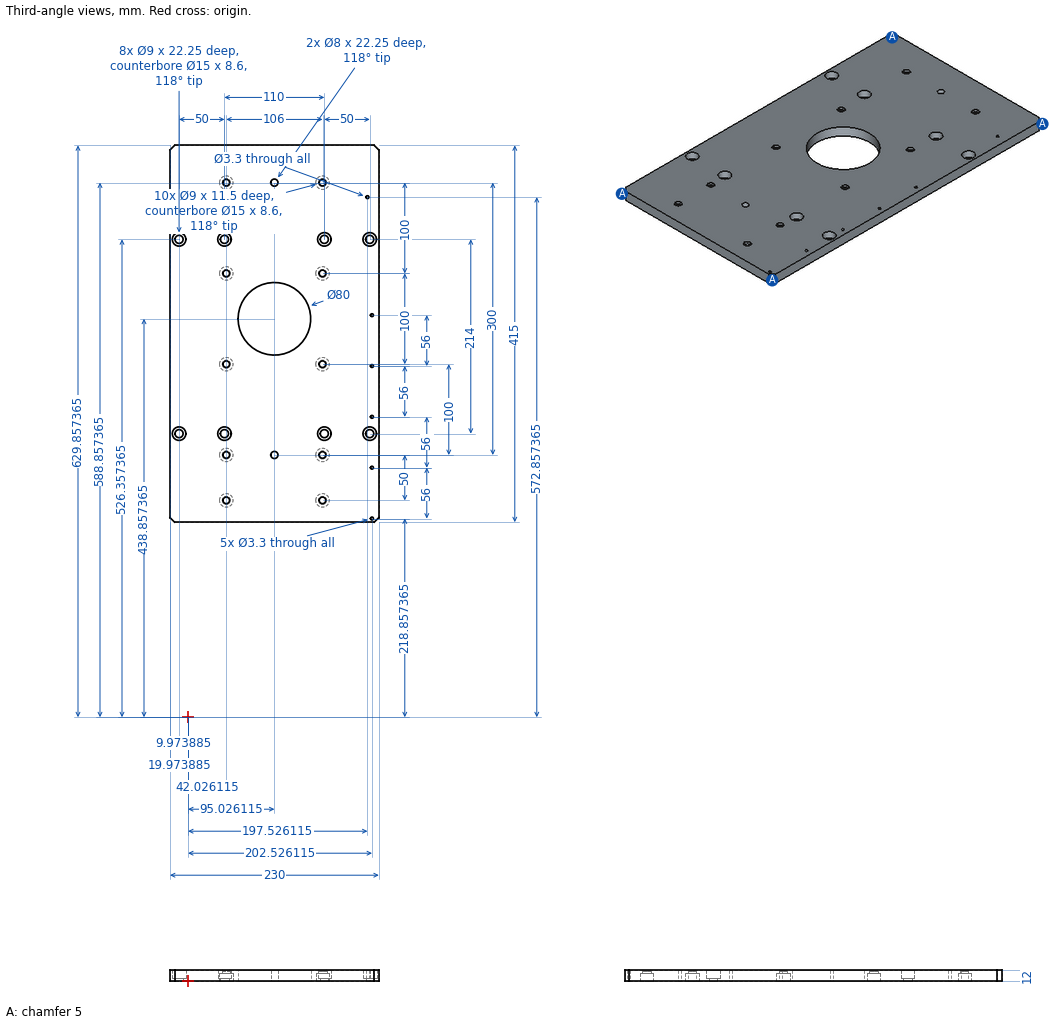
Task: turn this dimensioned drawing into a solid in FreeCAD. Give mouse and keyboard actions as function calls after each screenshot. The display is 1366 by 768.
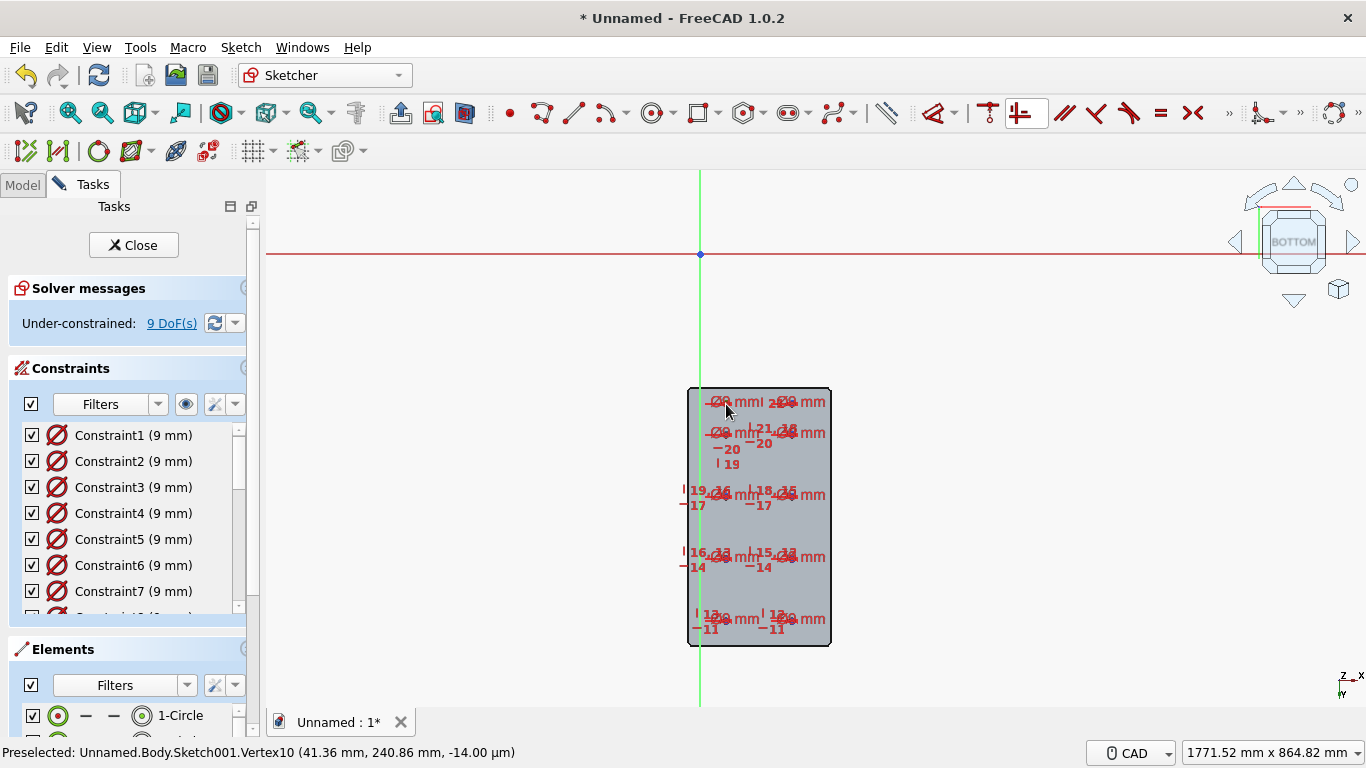
click(1042, 114)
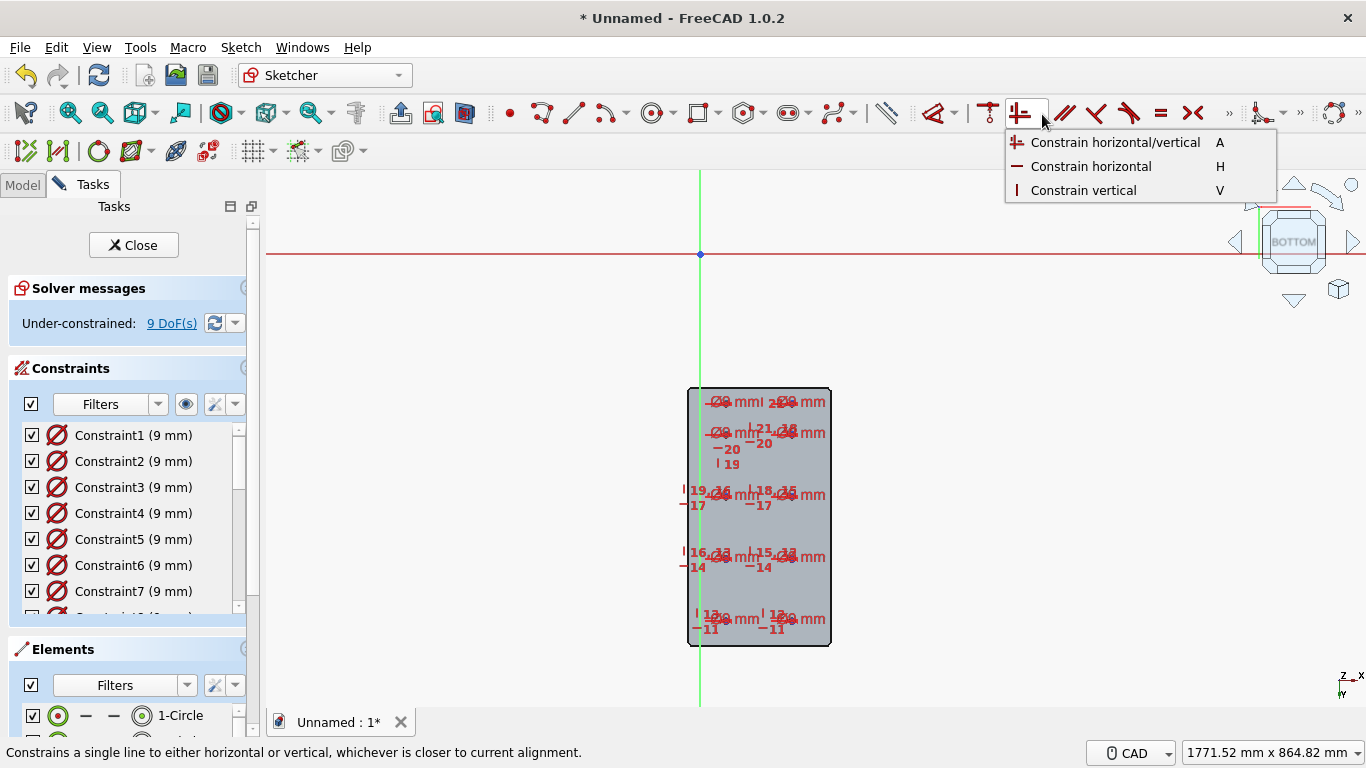
click(1141, 190)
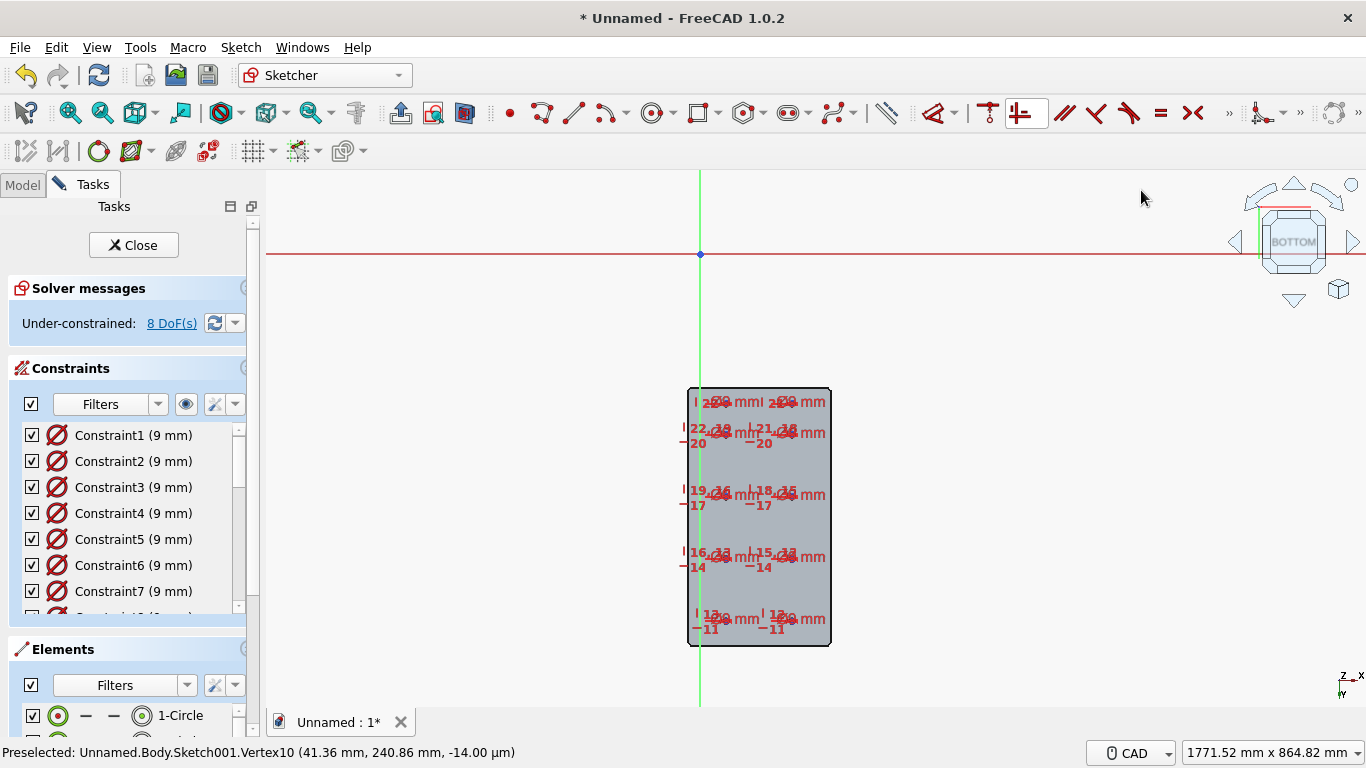
click(792, 404)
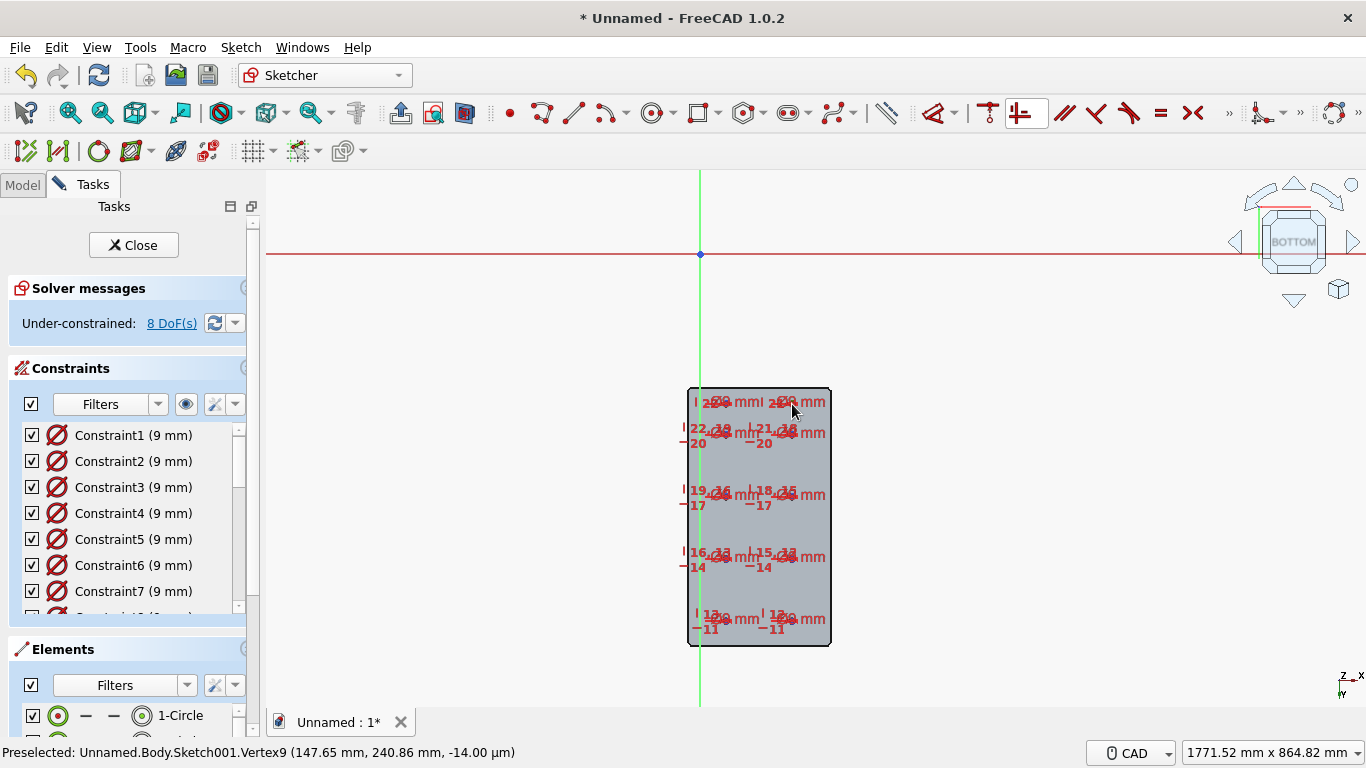
click(726, 404)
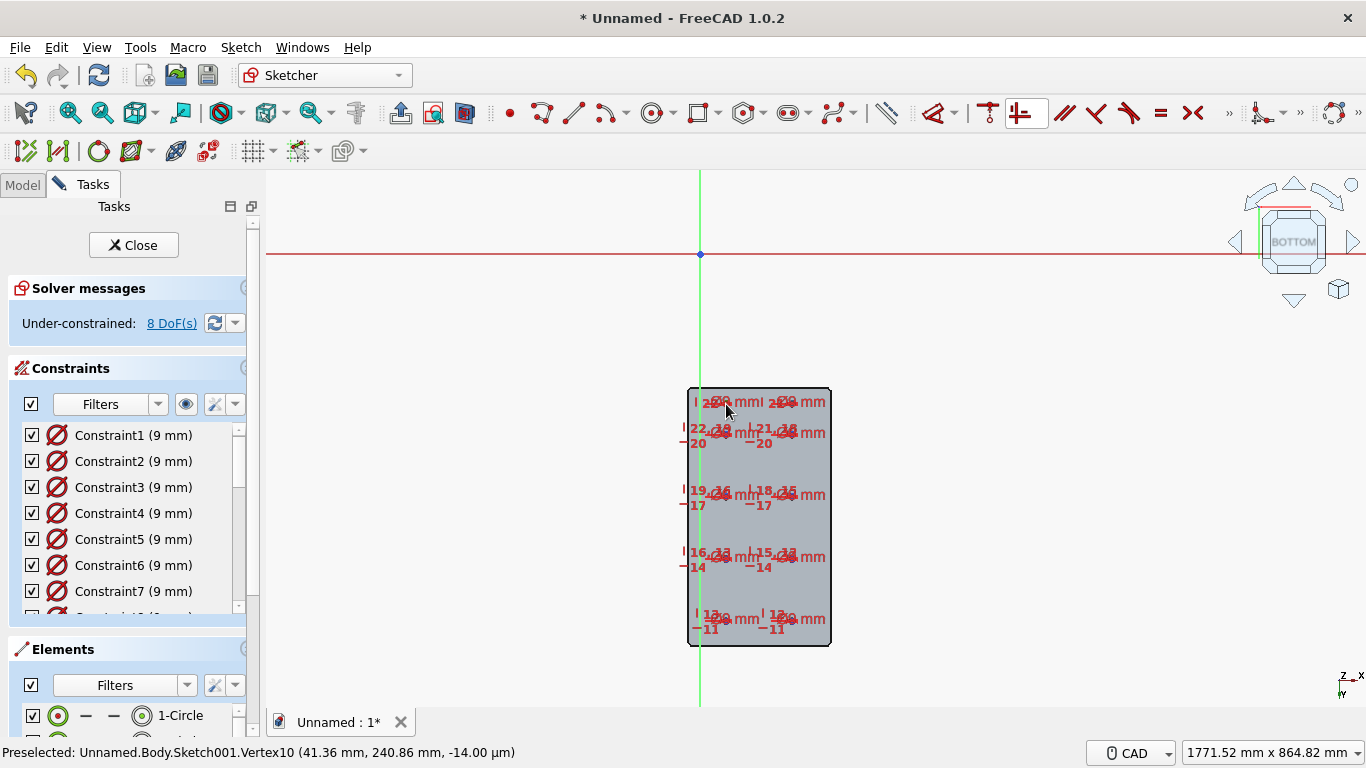
click(1042, 114)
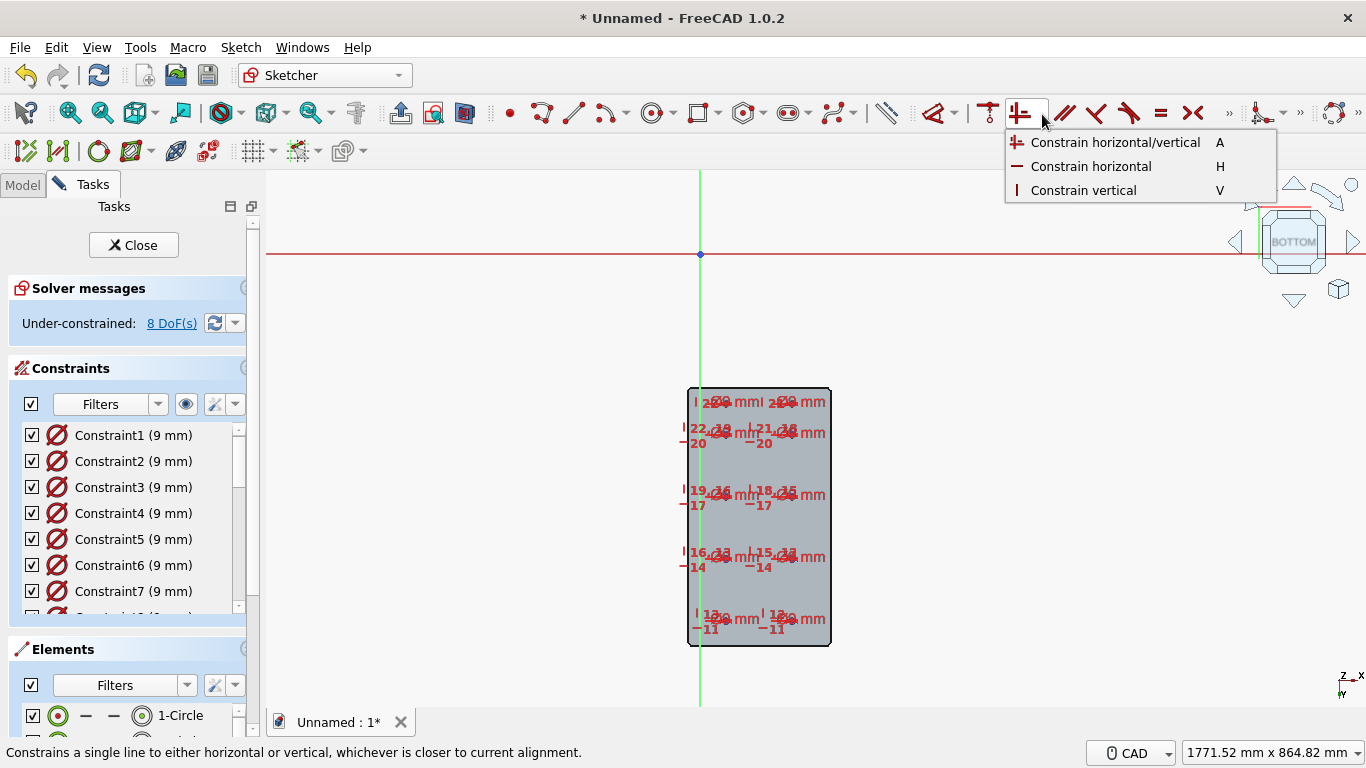
click(1141, 166)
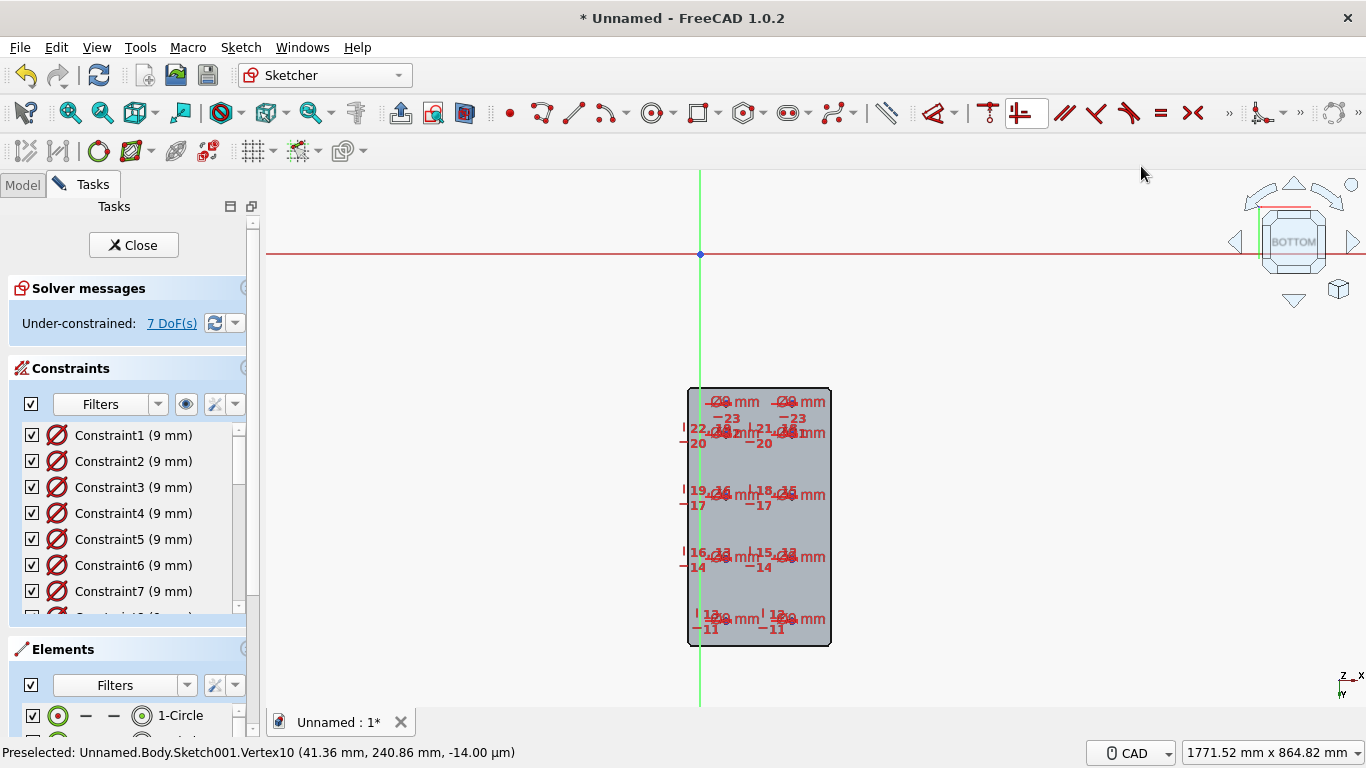
click(934, 114)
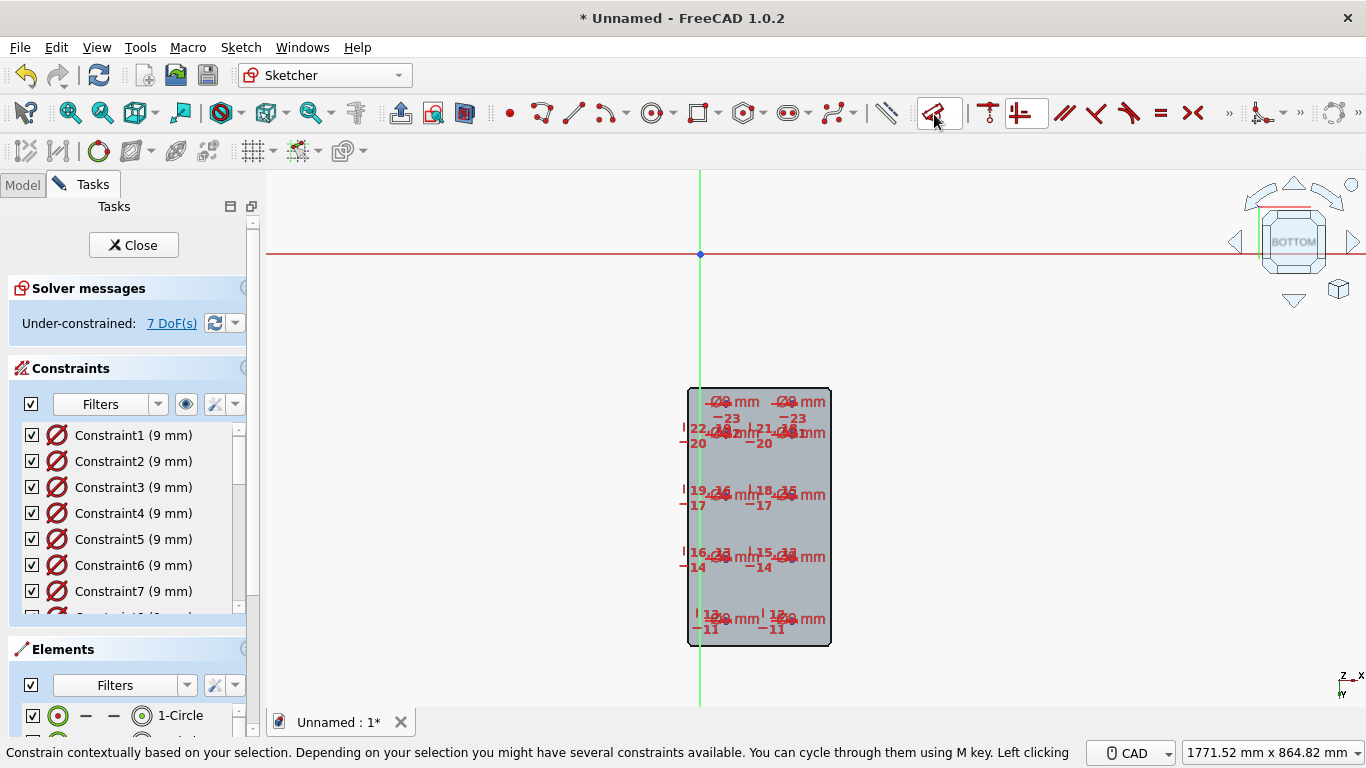
scroll(792, 435, up, 2)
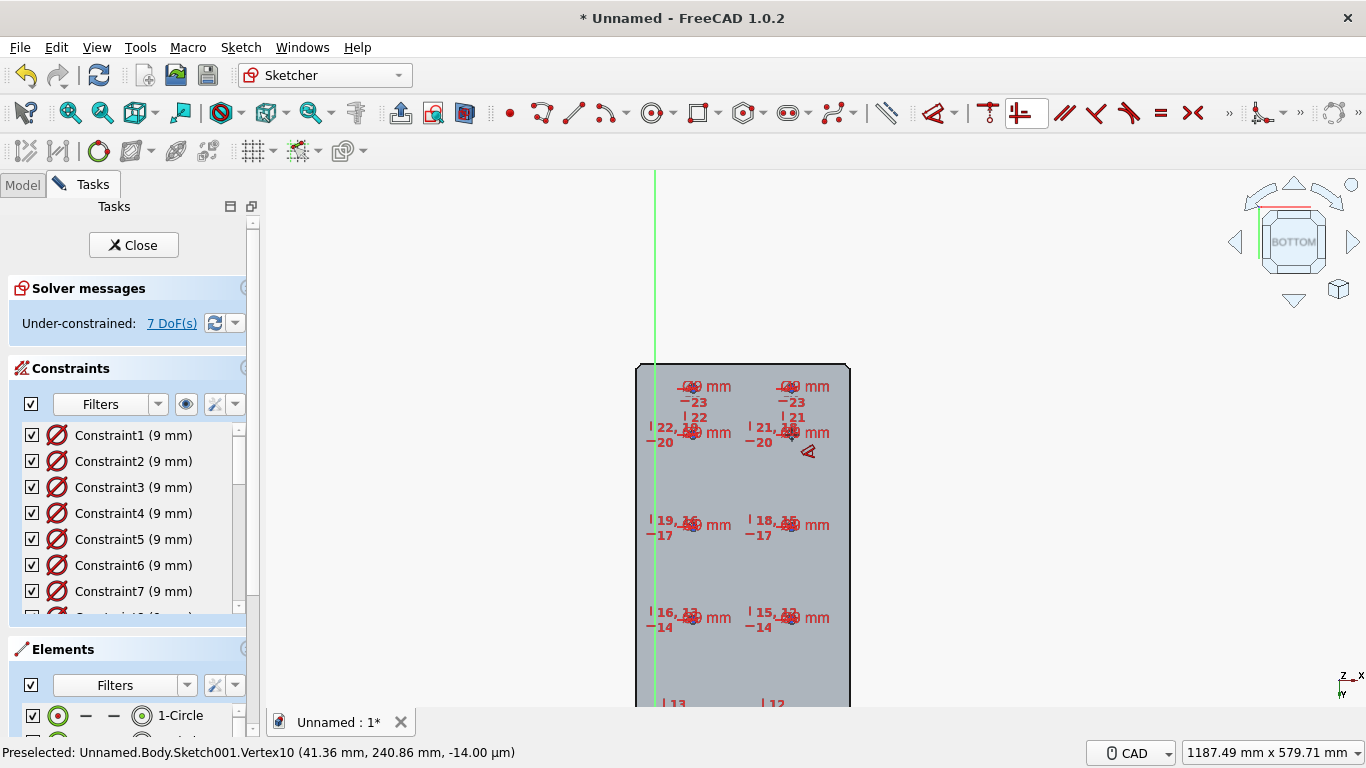
click(792, 435)